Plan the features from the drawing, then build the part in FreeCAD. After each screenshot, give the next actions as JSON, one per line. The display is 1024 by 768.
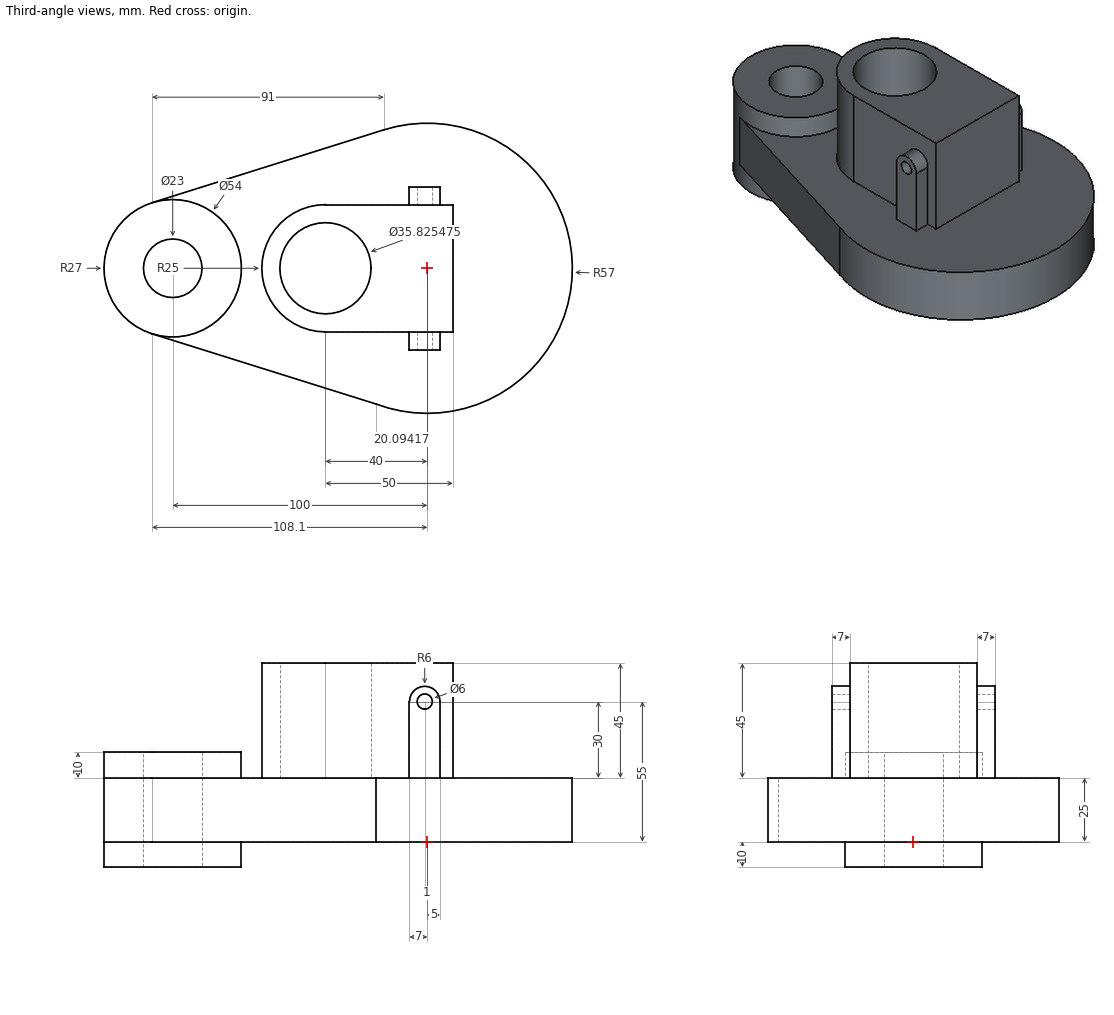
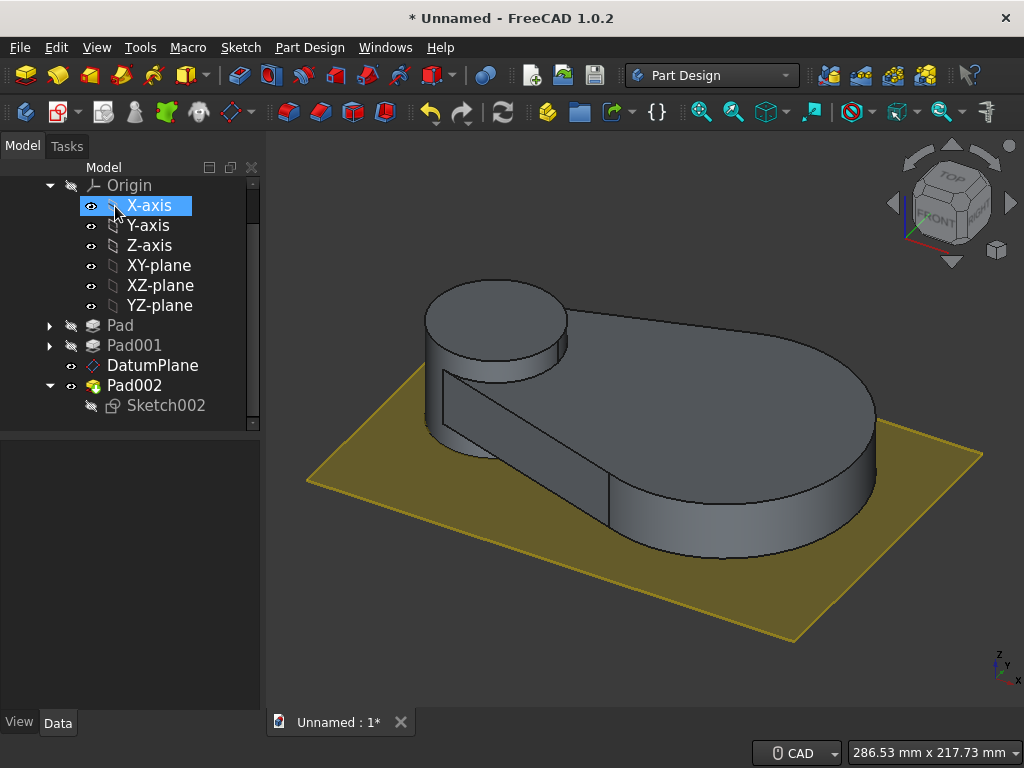
{"action": "left_click", "coordinate": [116, 366]}
{"action": "key", "text": "space"}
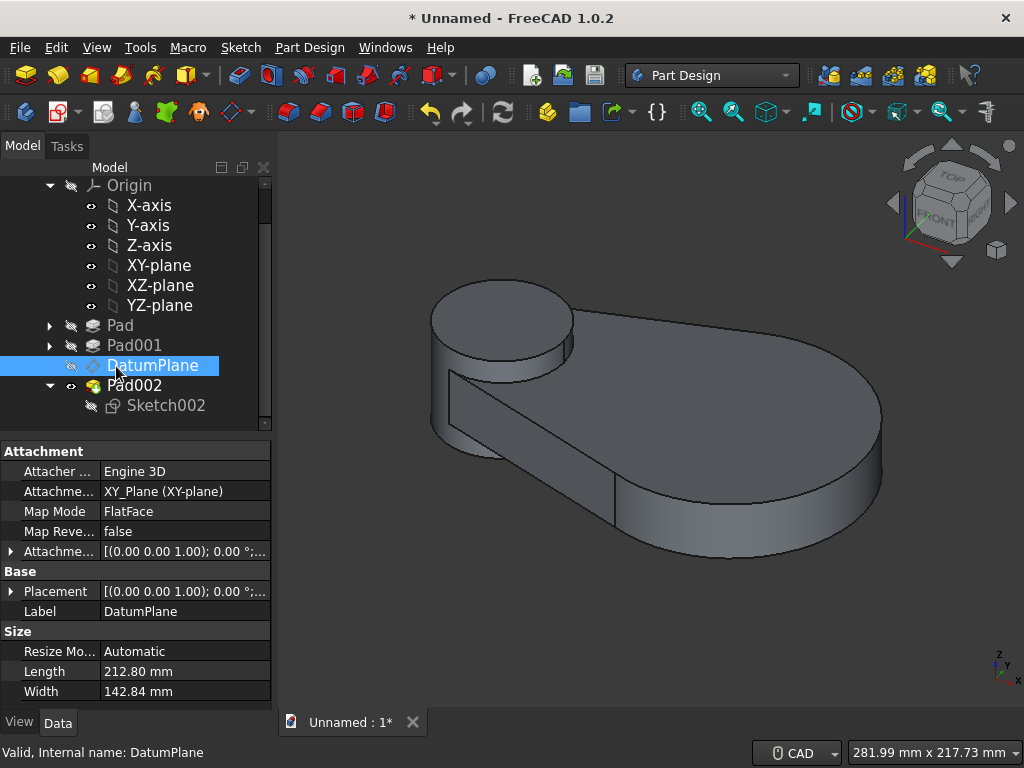
{"action": "left_click", "coordinate": [502, 319]}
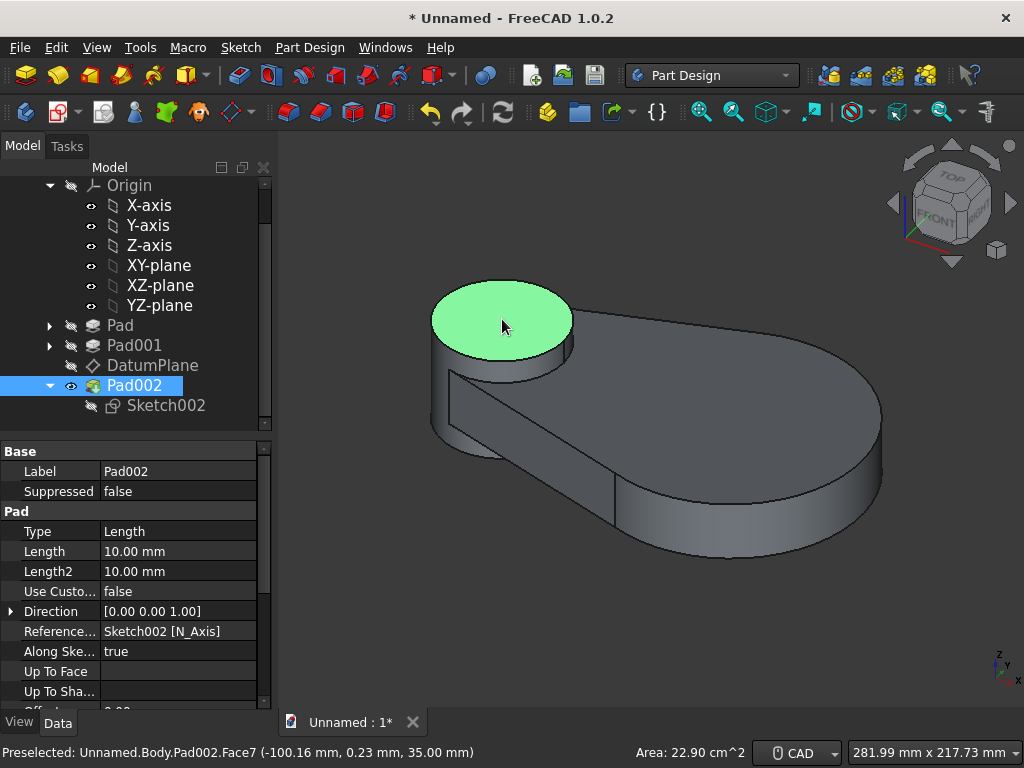
{"action": "left_click", "coordinate": [58, 112]}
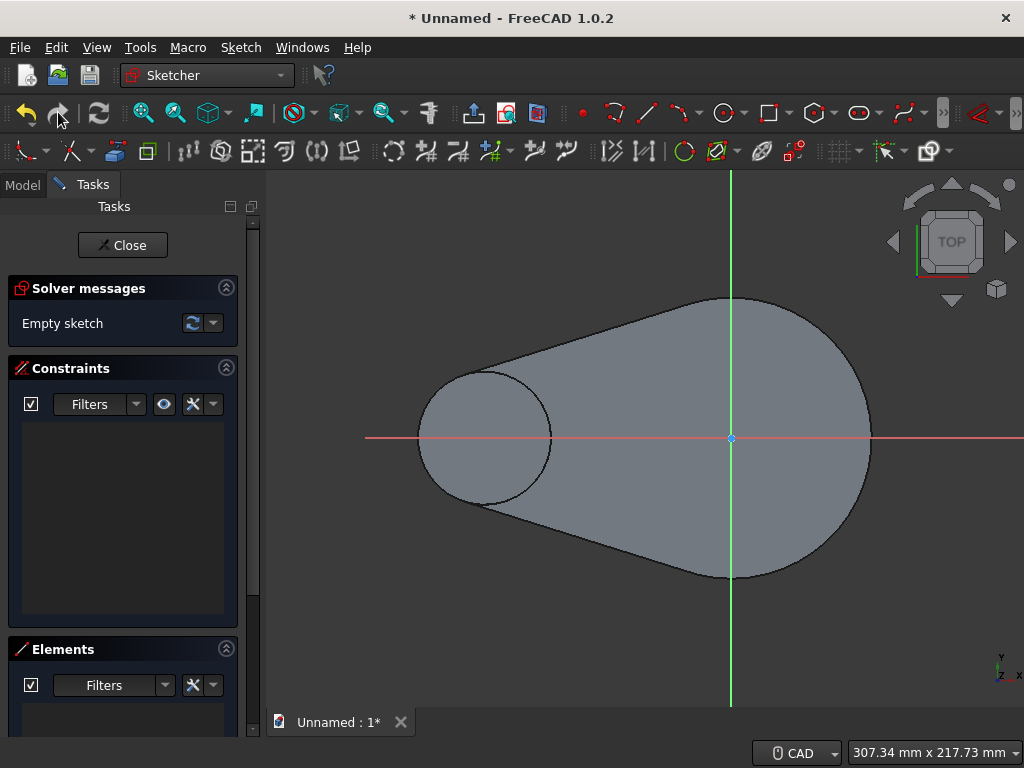
{"action": "scroll", "coordinate": [466, 438], "scroll_direction": "up", "scroll_amount": 9}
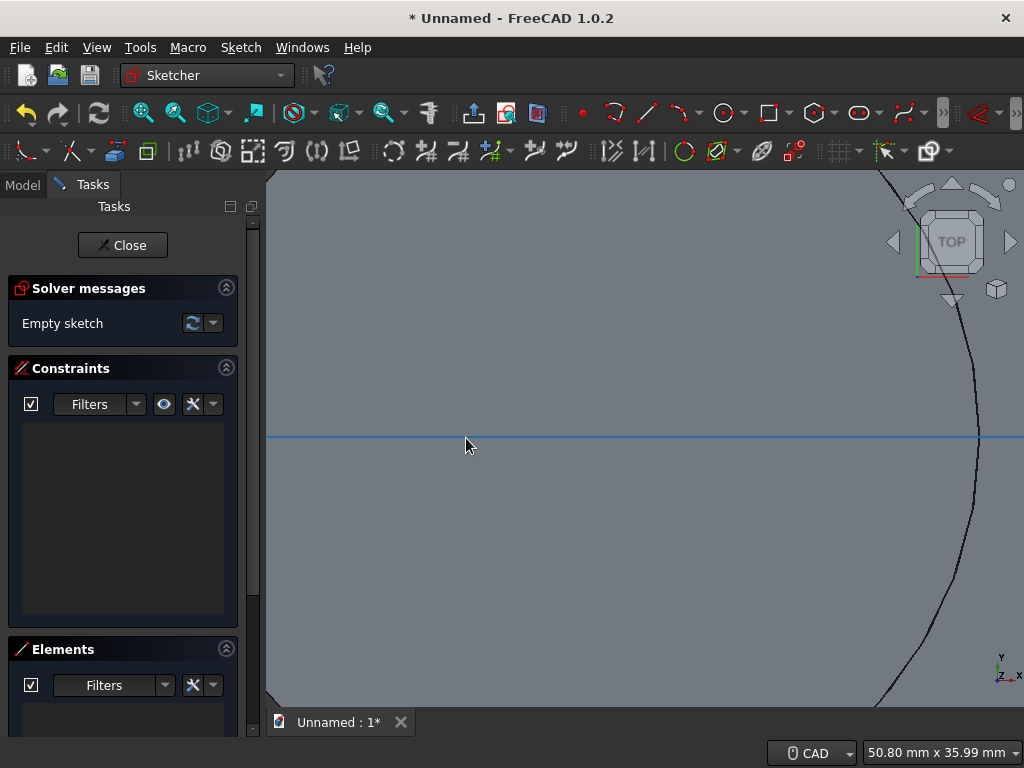
{"action": "key", "text": "g c"}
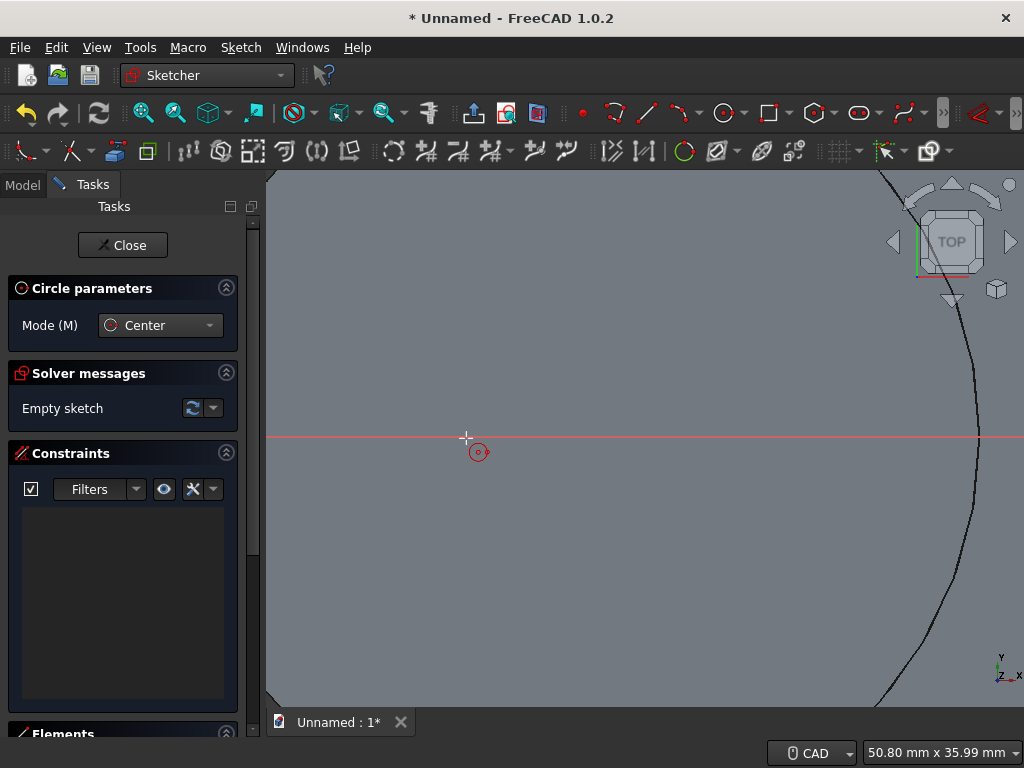
{"action": "left_click", "coordinate": [577, 437]}
{"action": "left_click", "coordinate": [698, 315]}
{"action": "key", "text": "Escape"}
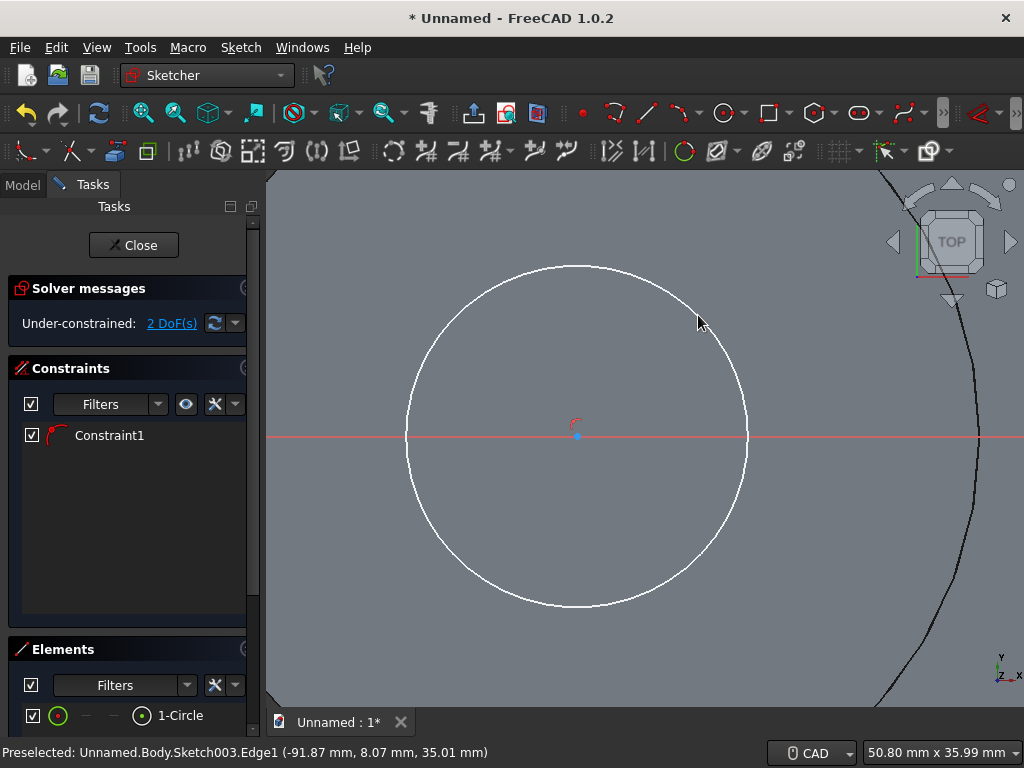
{"action": "key", "text": "d"}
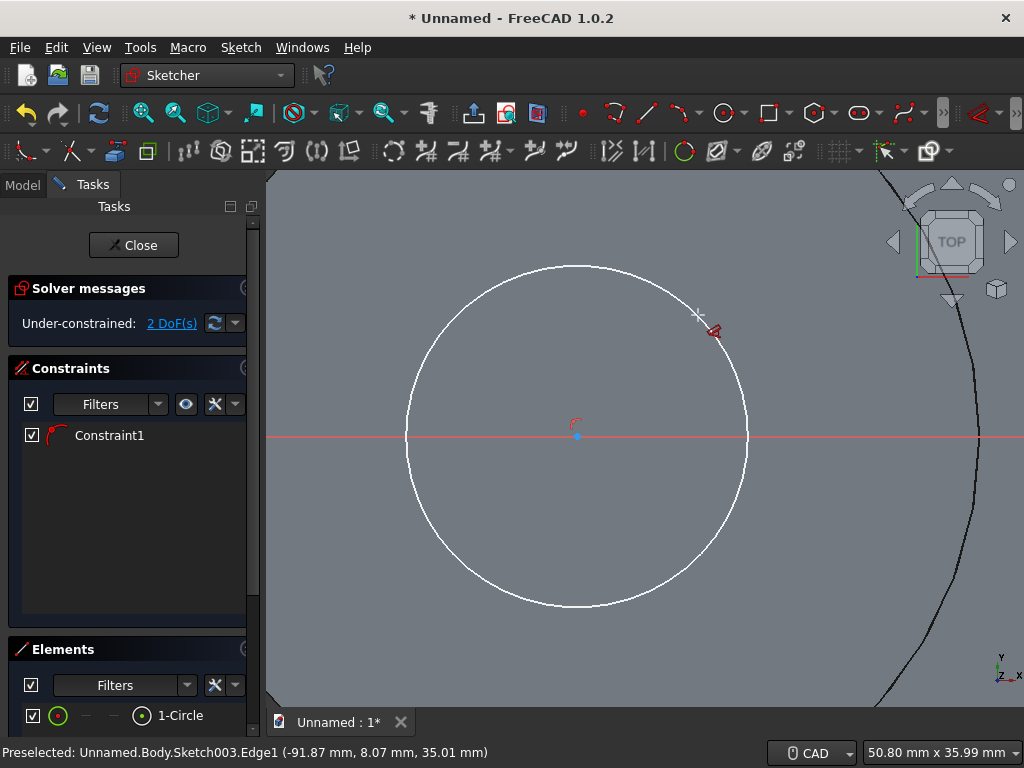
{"action": "left_click", "coordinate": [697, 315]}
{"action": "left_click", "coordinate": [719, 292]}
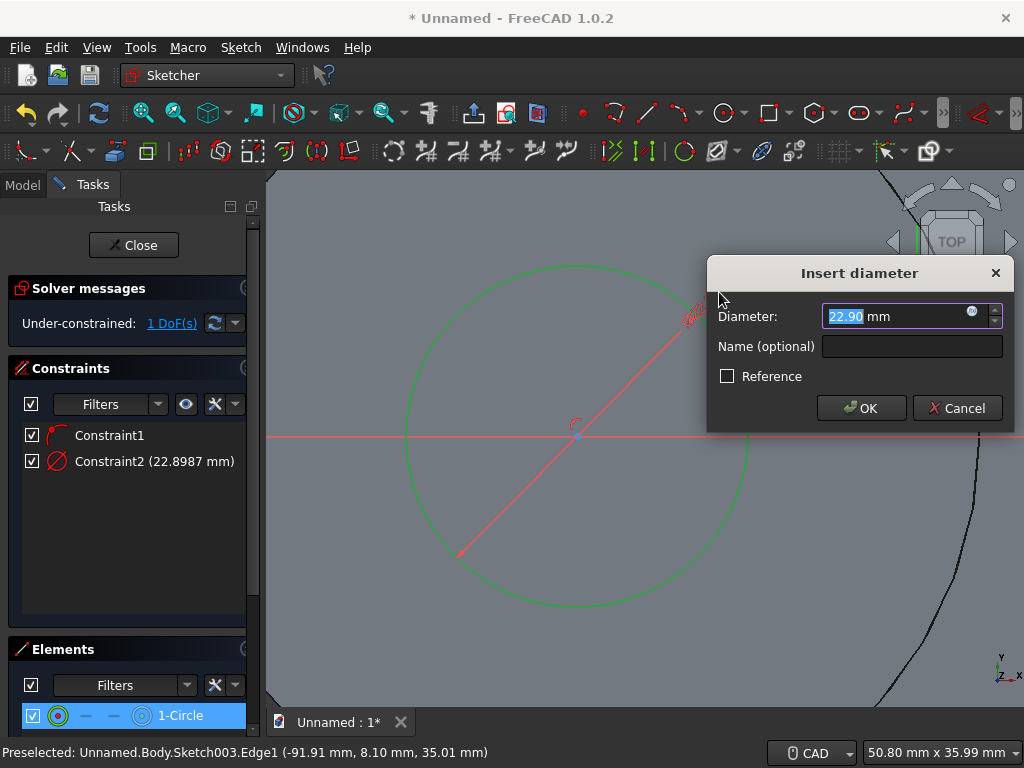
{"action": "type", "text": "23"}
{"action": "key", "text": "Return"}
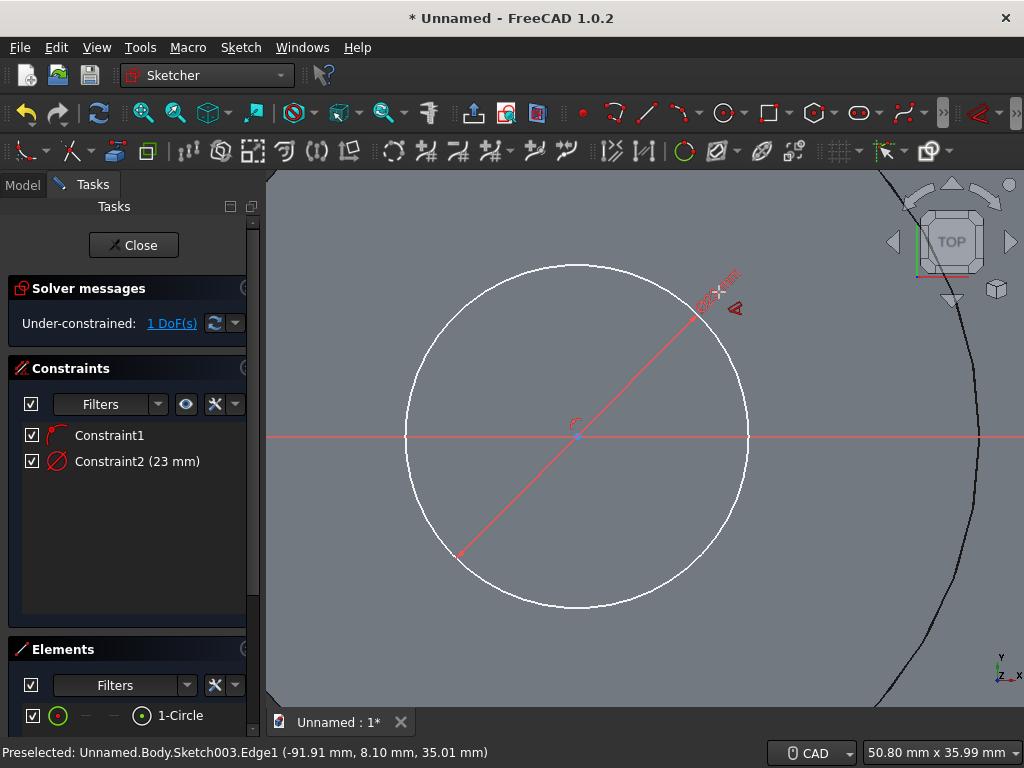
{"action": "left_click", "coordinate": [577, 437]}
{"action": "left_click", "coordinate": [718, 471]}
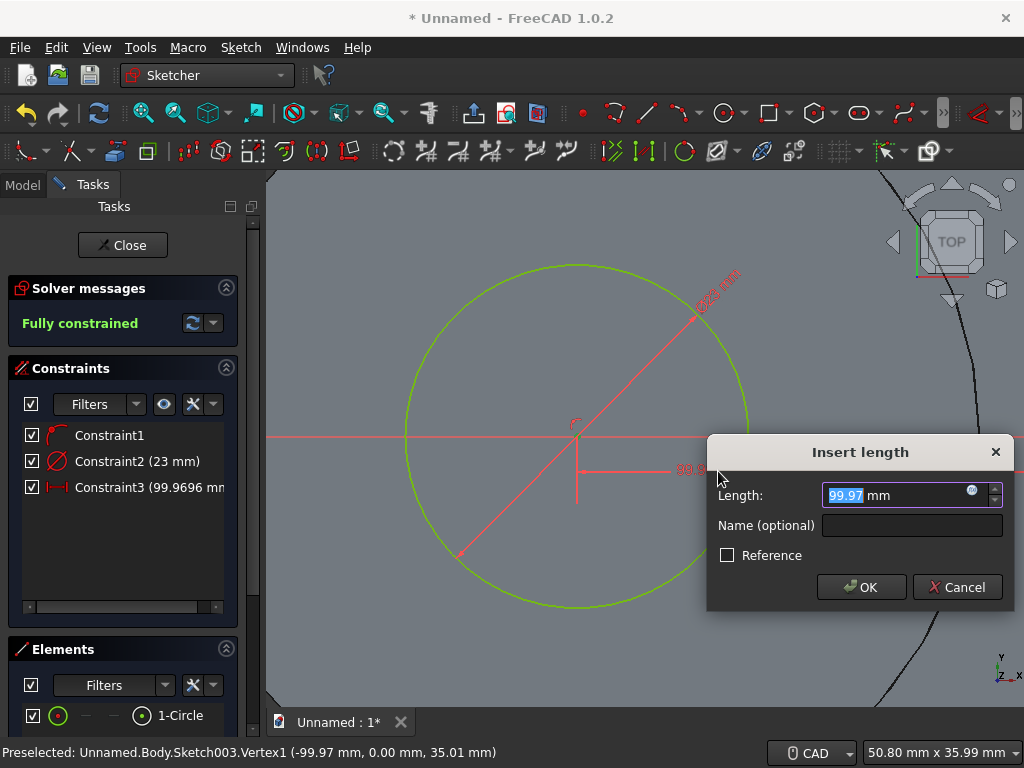
{"action": "type", "text": "100"}
{"action": "key", "text": "Return"}
{"action": "key", "text": "Escape"}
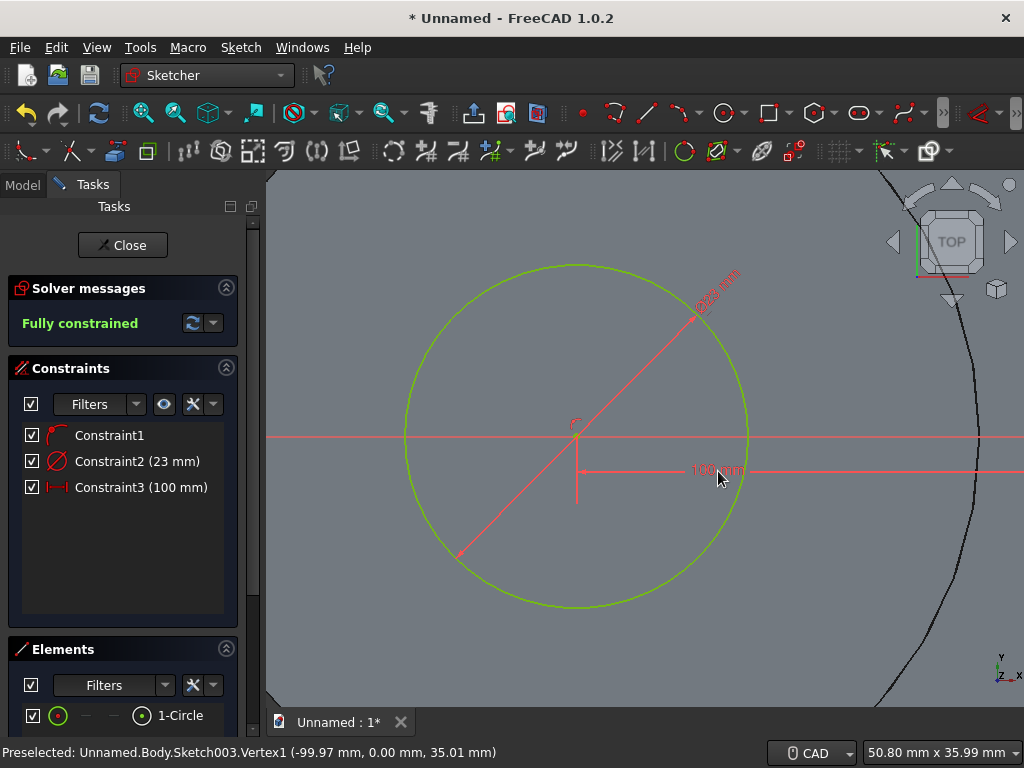
{"action": "left_click", "coordinate": [123, 245]}